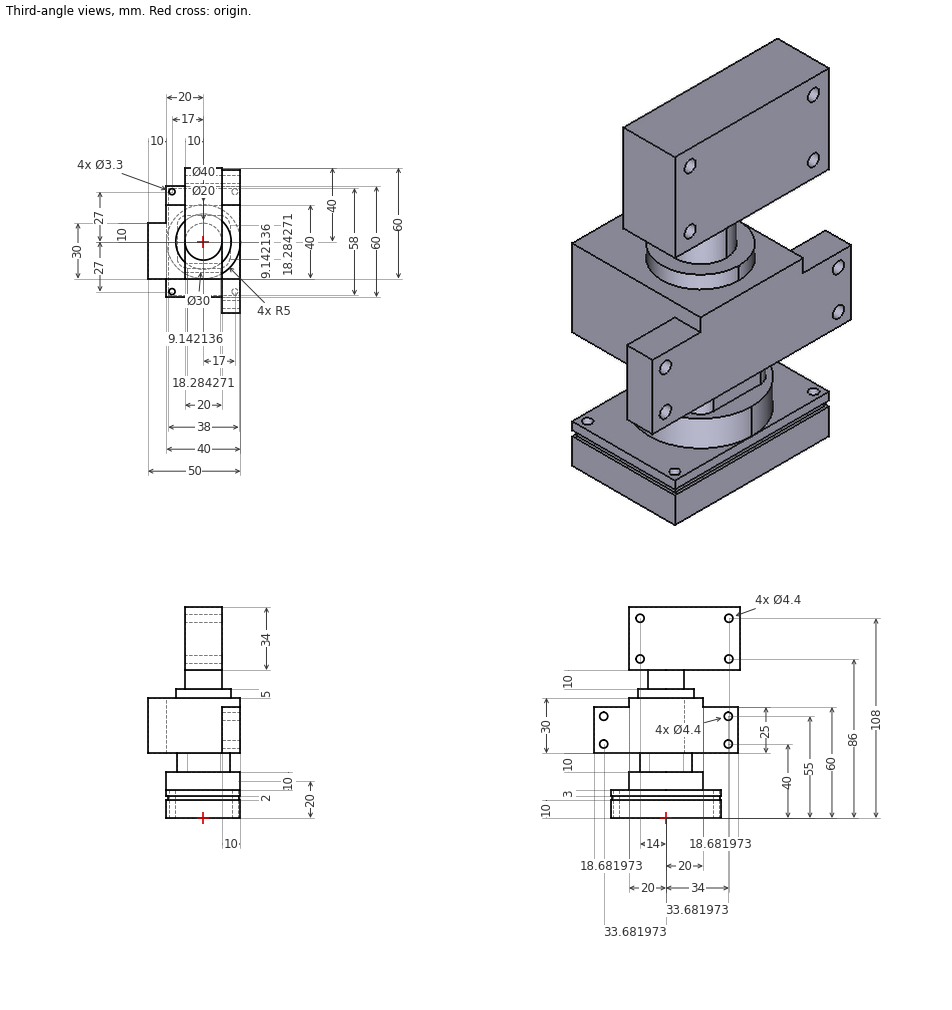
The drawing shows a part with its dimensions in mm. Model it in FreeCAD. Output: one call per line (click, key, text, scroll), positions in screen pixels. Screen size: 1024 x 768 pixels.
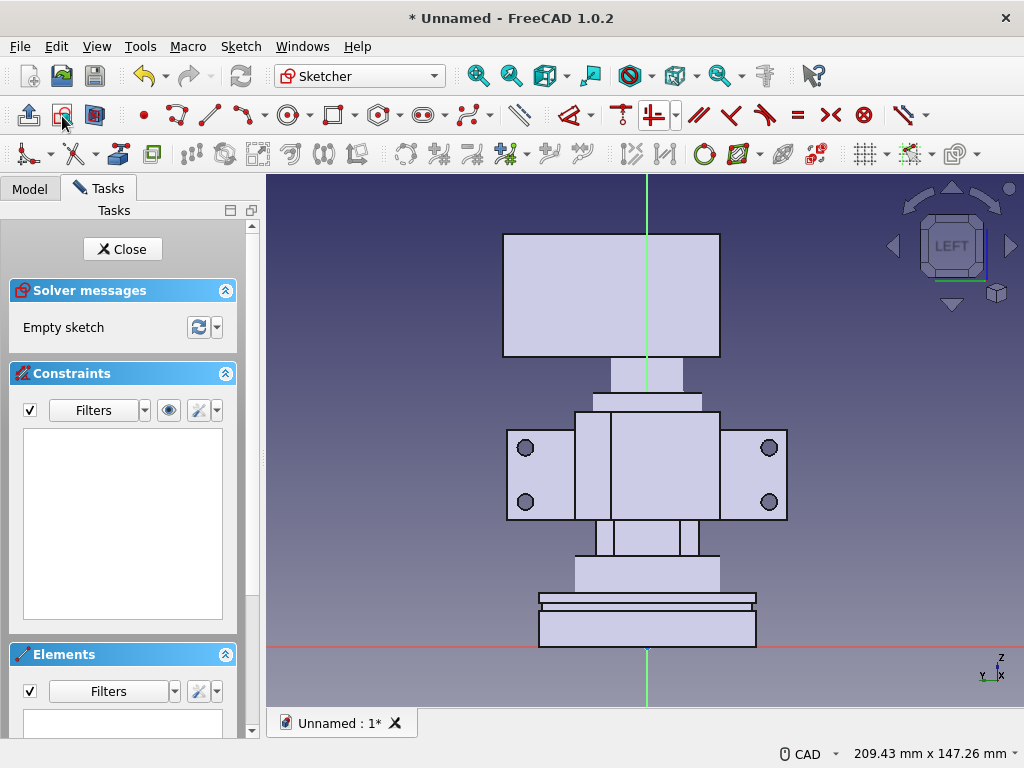
key(g)
key(c)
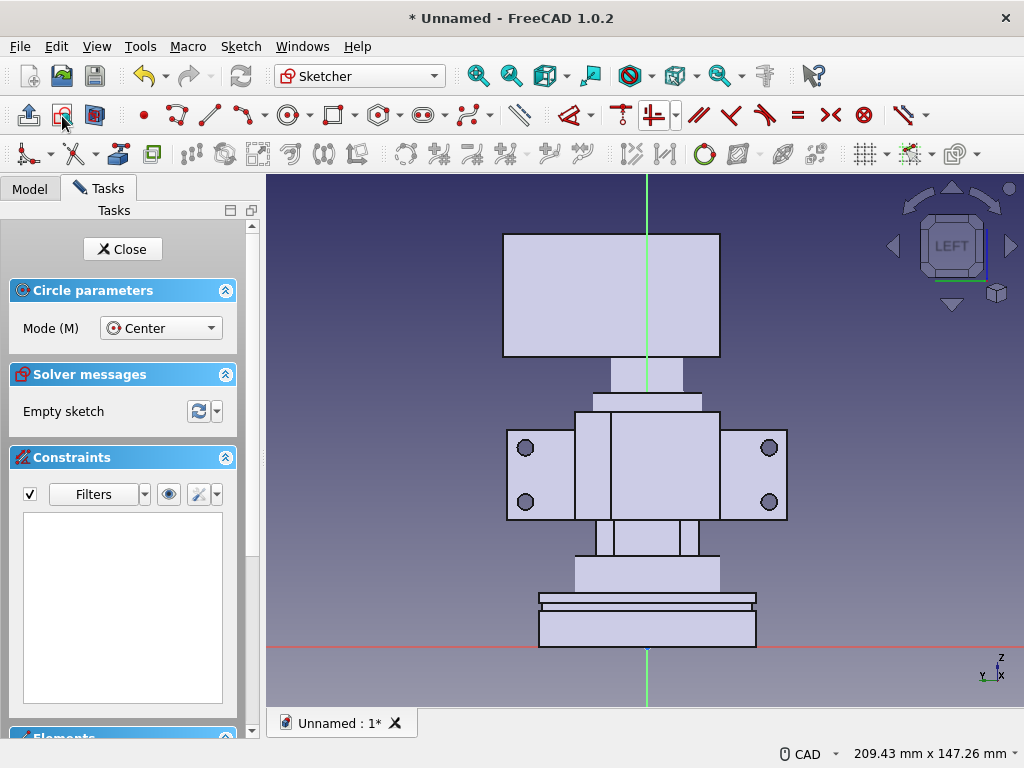
scroll(524, 256, up, 6)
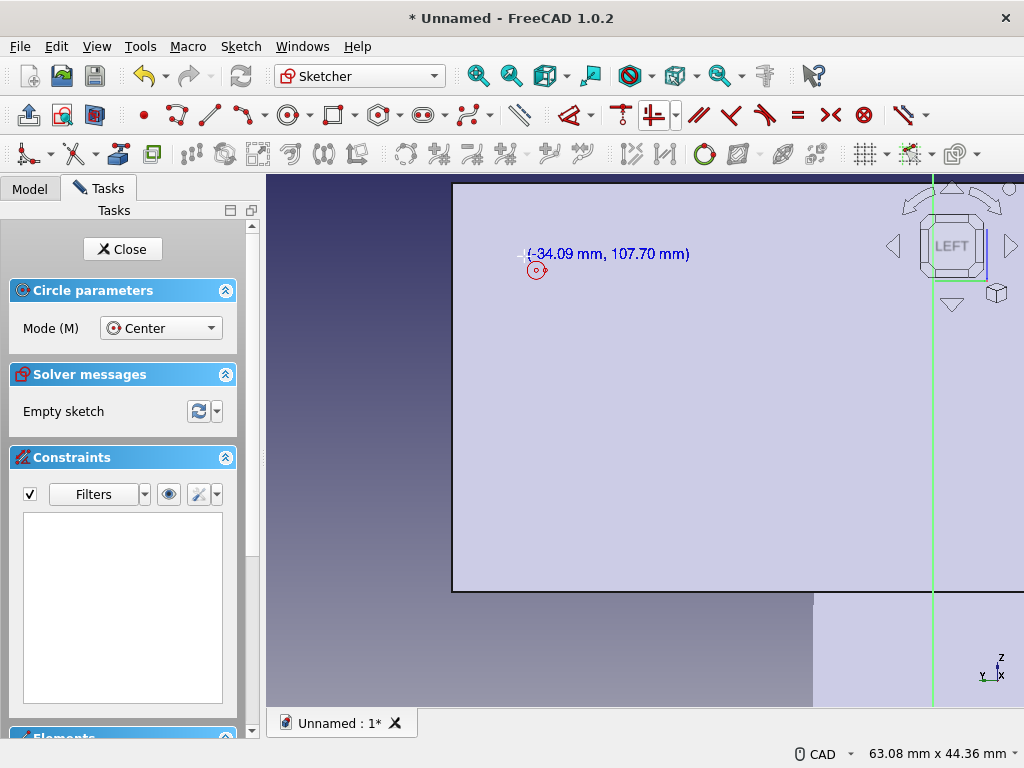
click(524, 255)
move(543, 237)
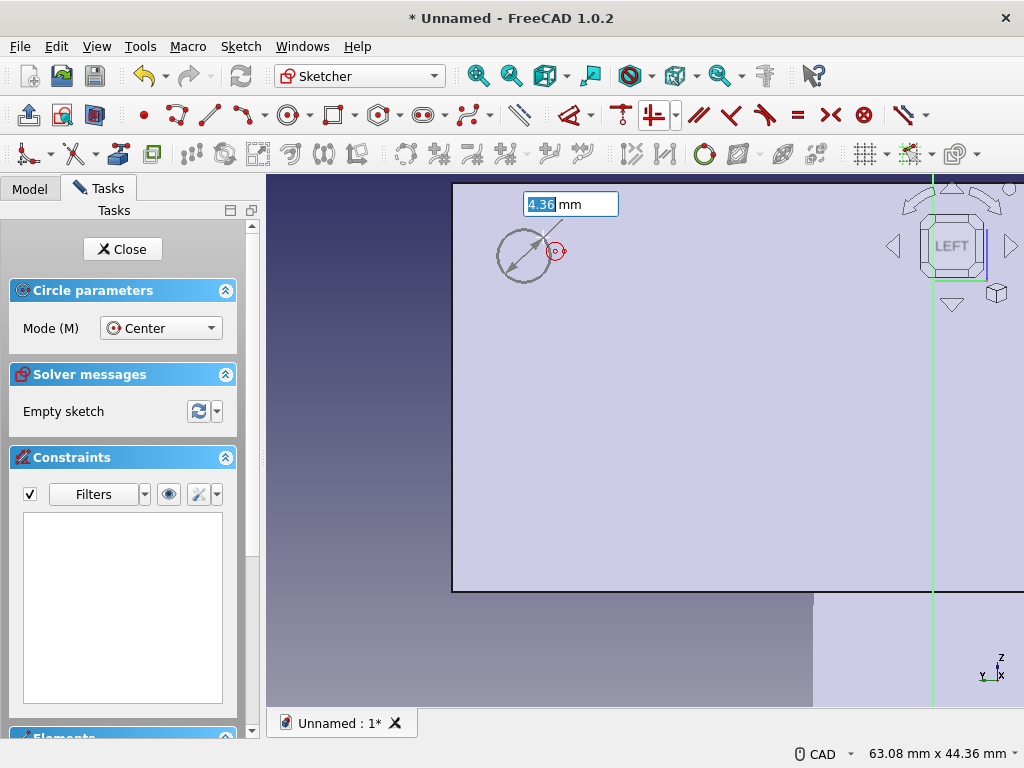
text(4.4)
key(Return)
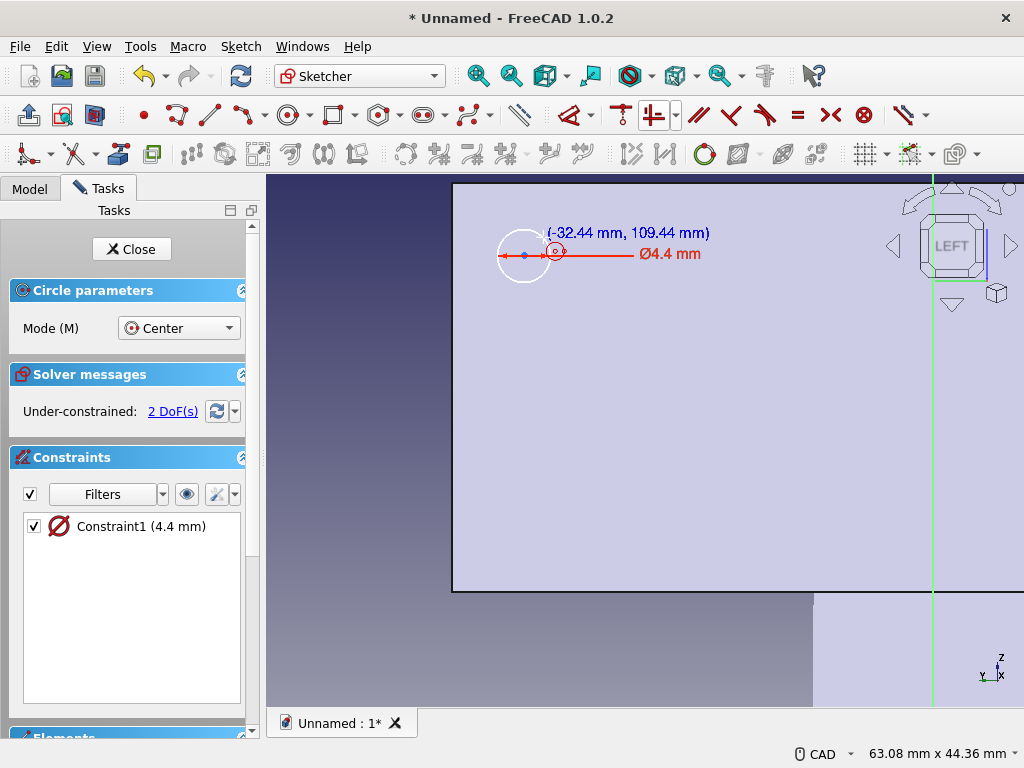
click(524, 520)
move(543, 501)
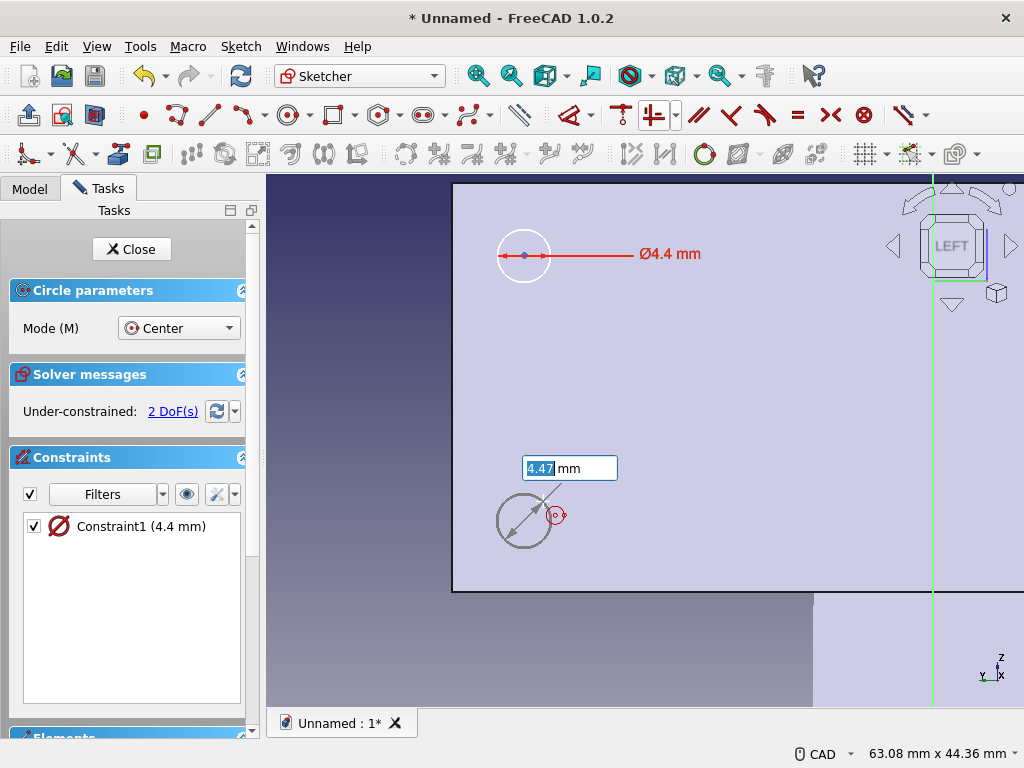
text(4.4)
key(Return)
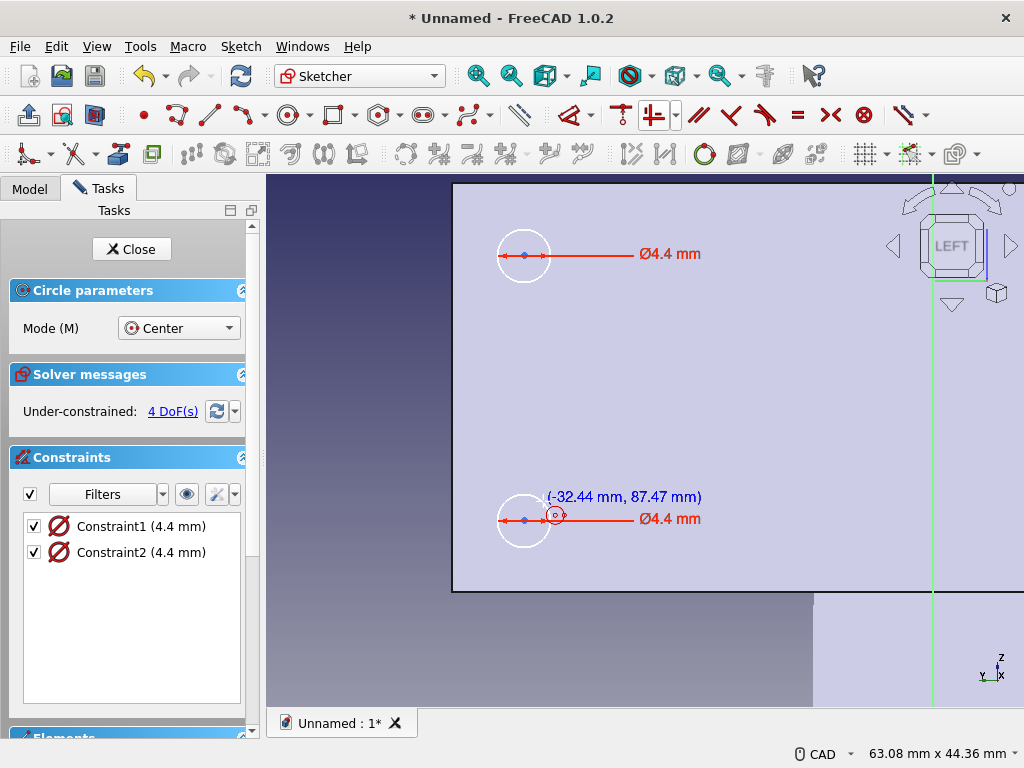
scroll(499, 293, down, 7)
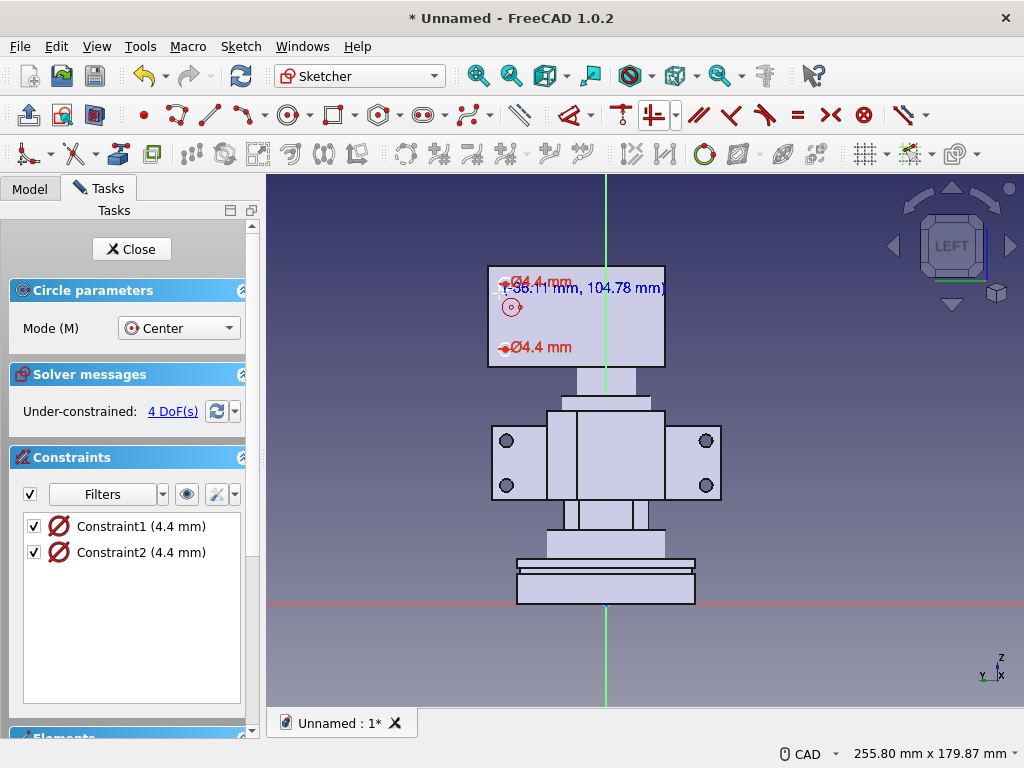
scroll(648, 284, up, 7)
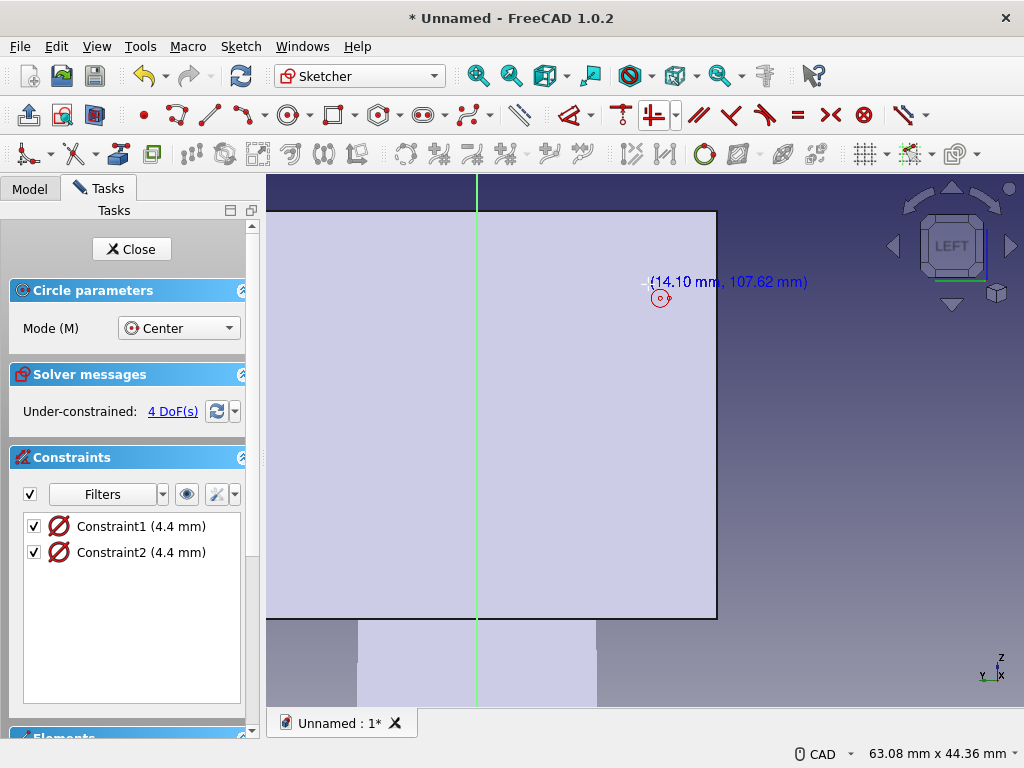
click(645, 283)
move(664, 264)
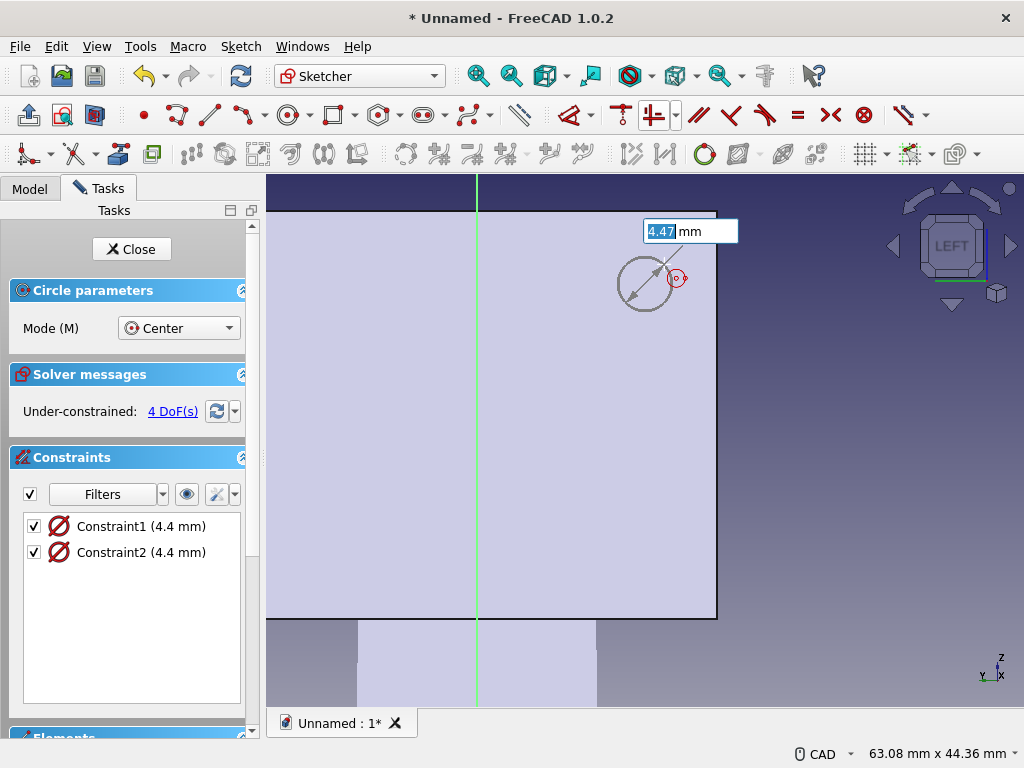
text(4.4)
key(Return)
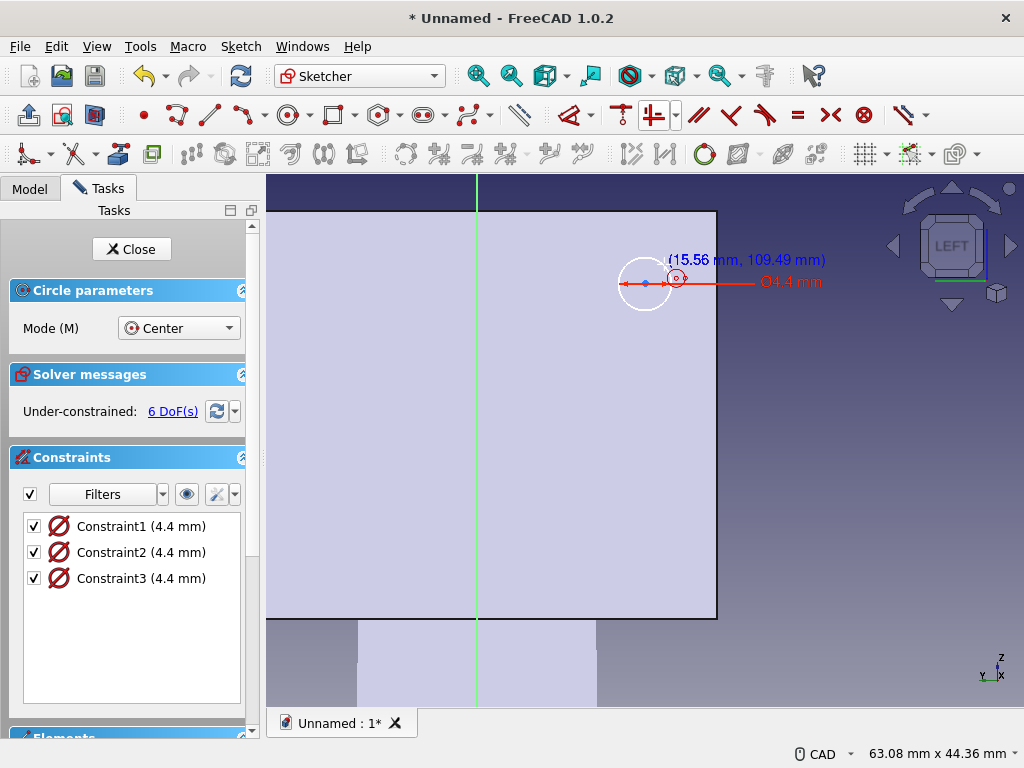
click(645, 547)
move(664, 529)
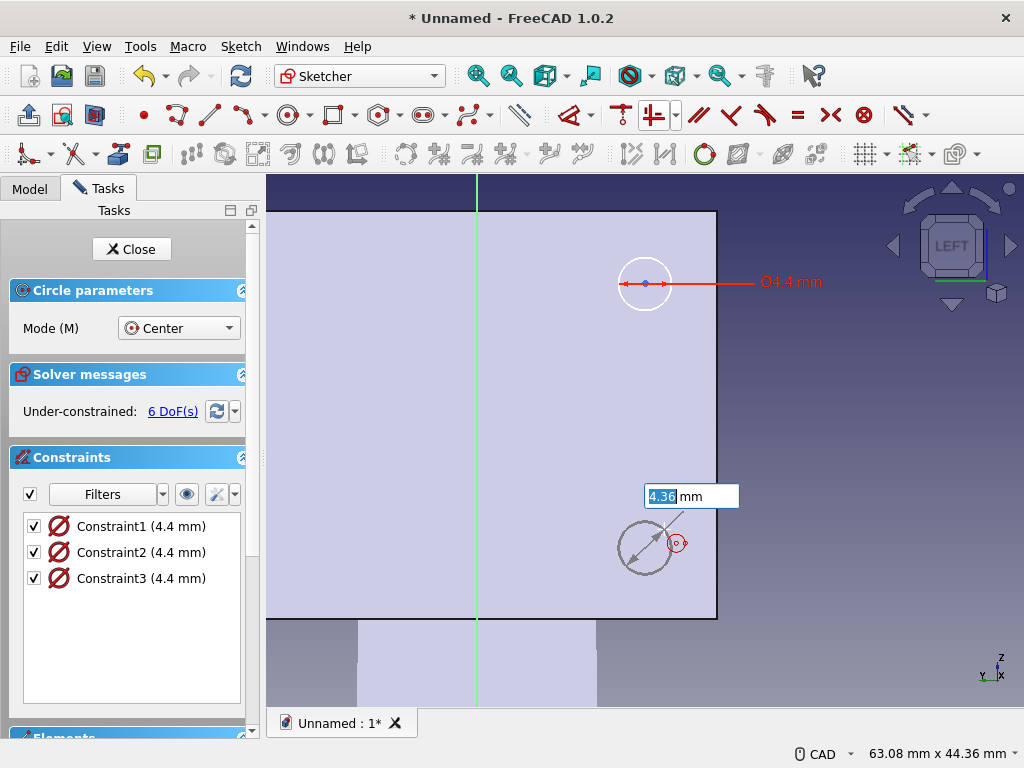
text(4.4)
key(Return)
key(Escape)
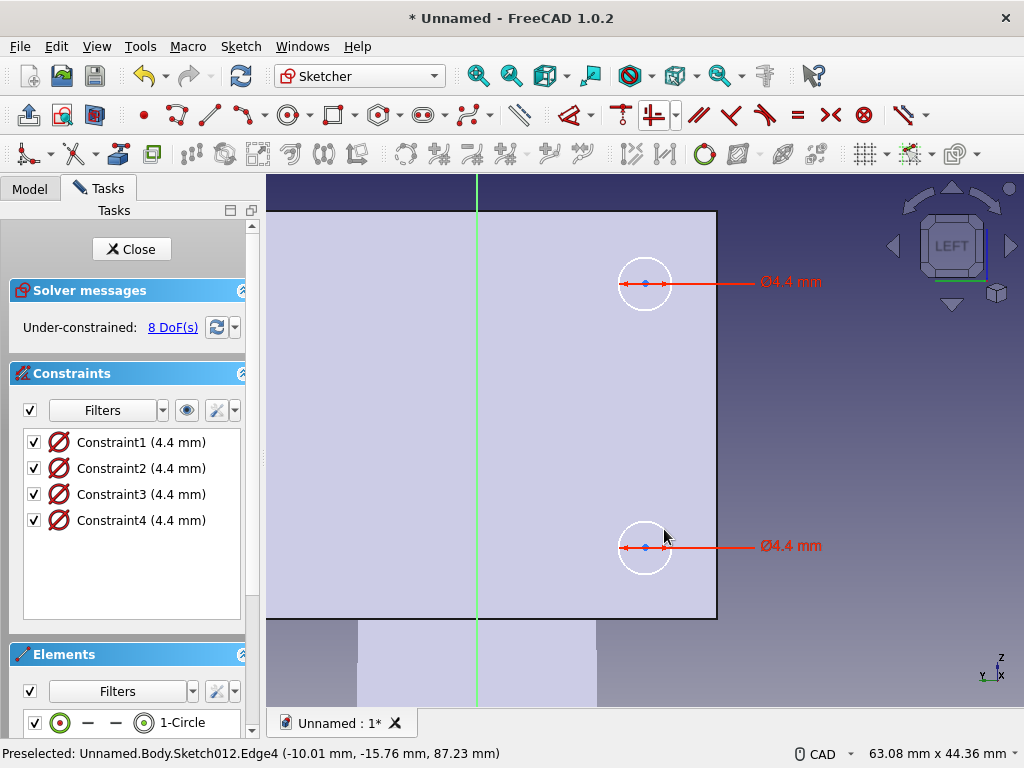
scroll(648, 284, down, 7)